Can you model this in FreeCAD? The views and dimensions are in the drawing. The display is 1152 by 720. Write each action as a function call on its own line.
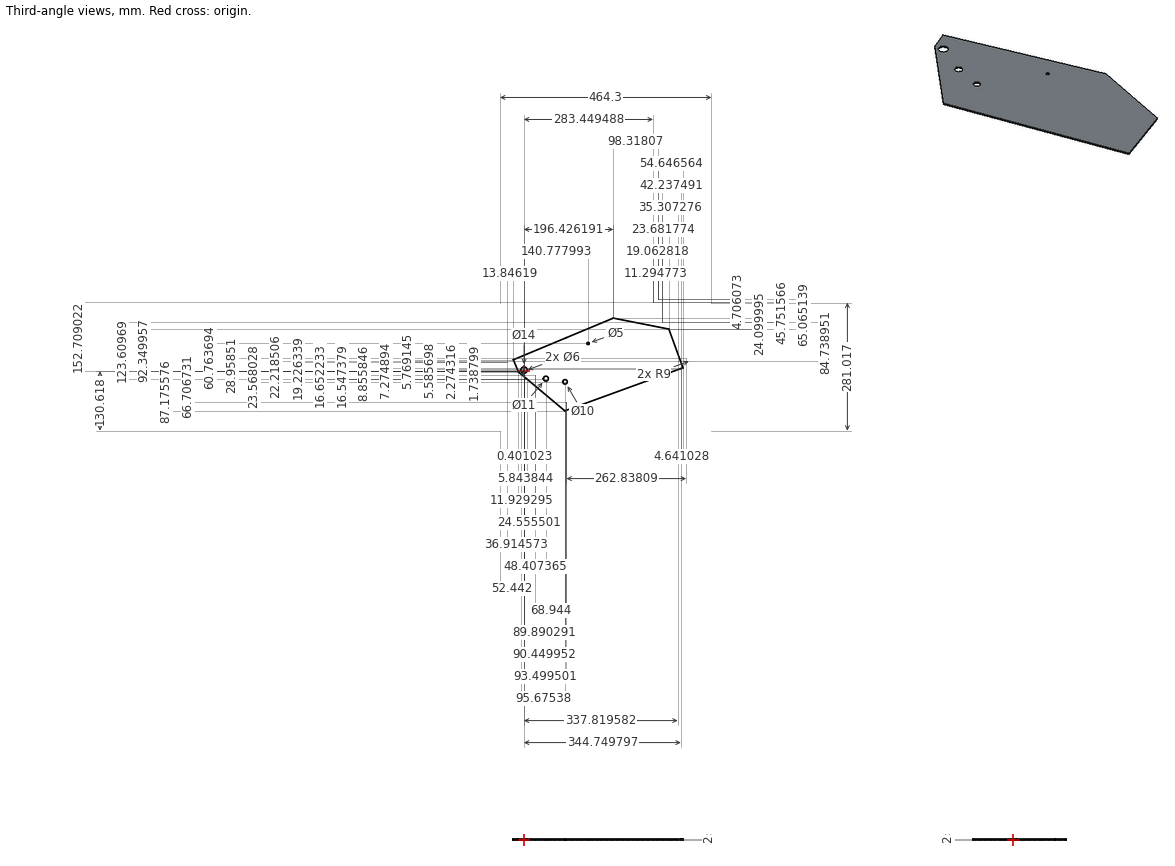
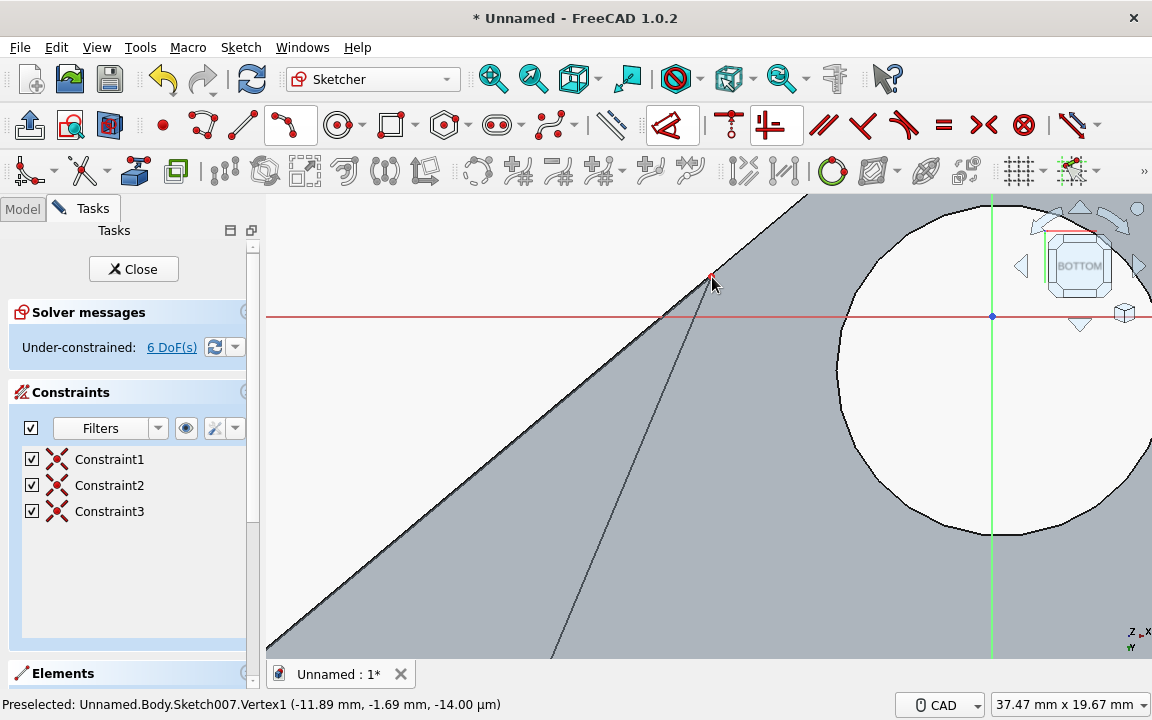
click(711, 277)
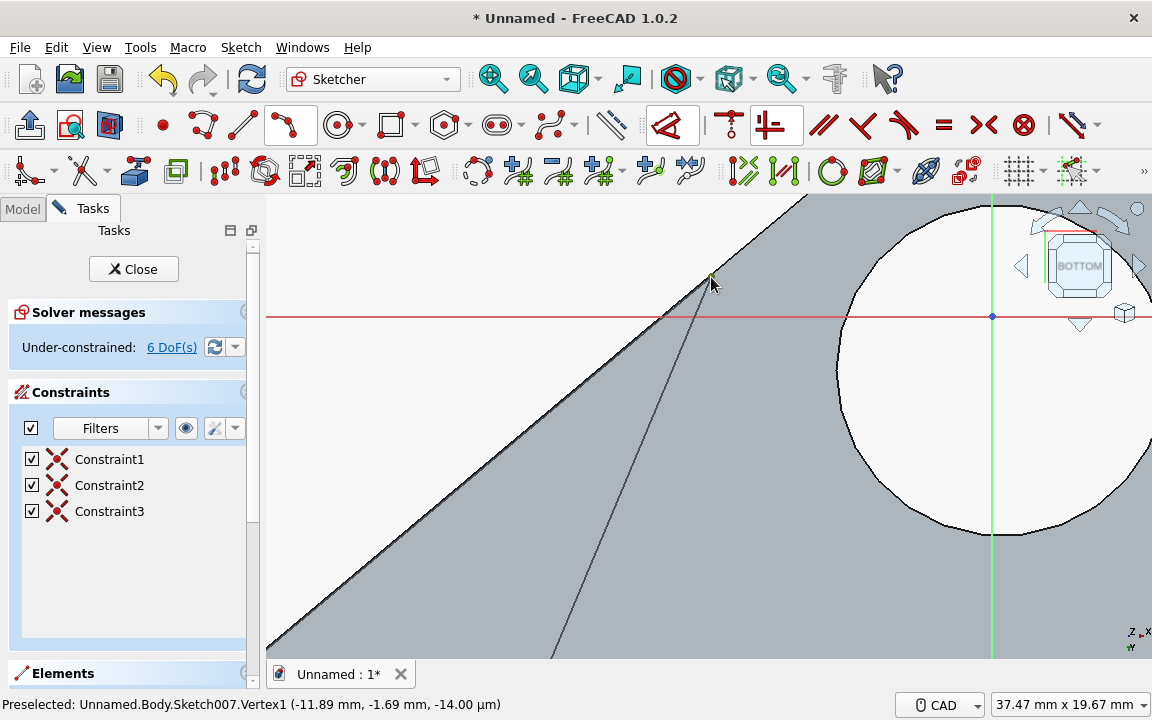
key(i)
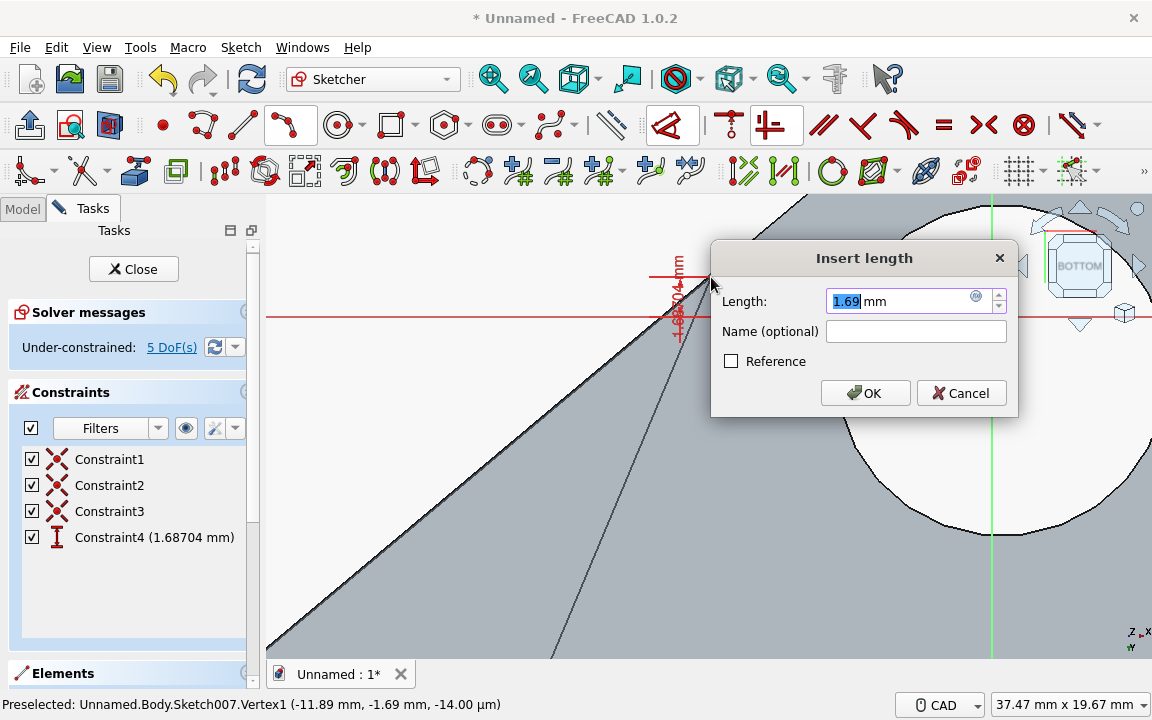
text(1.738799)
key(Return)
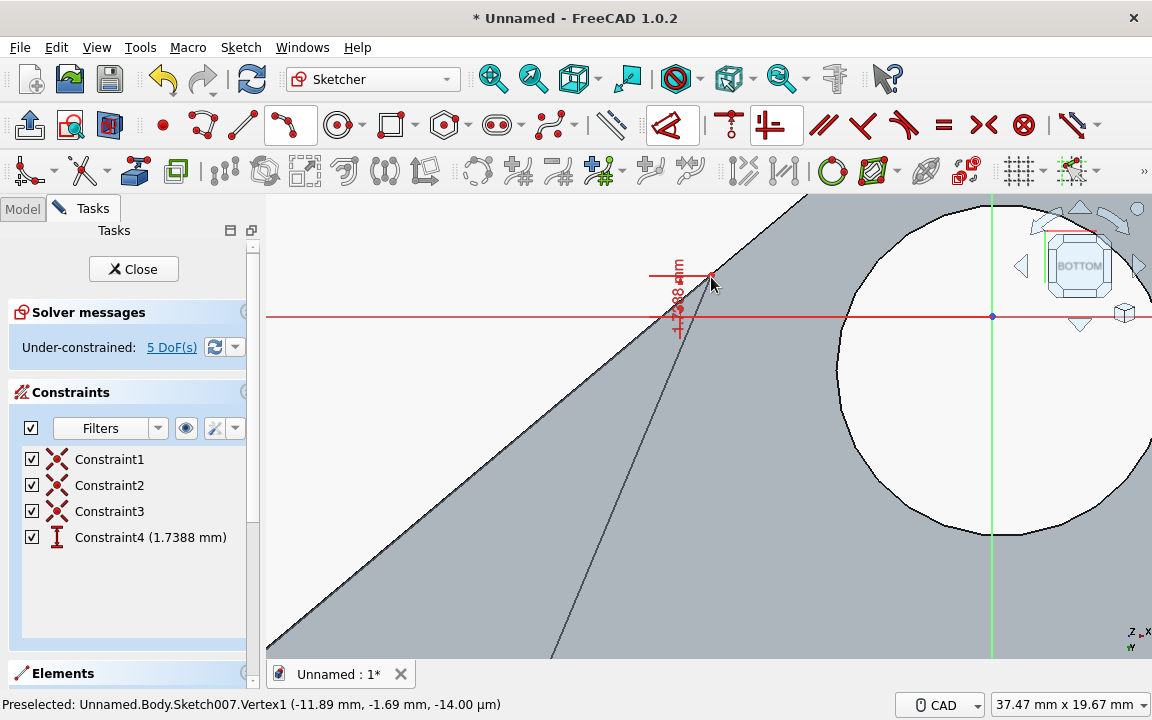
scroll(709, 292, down, 4)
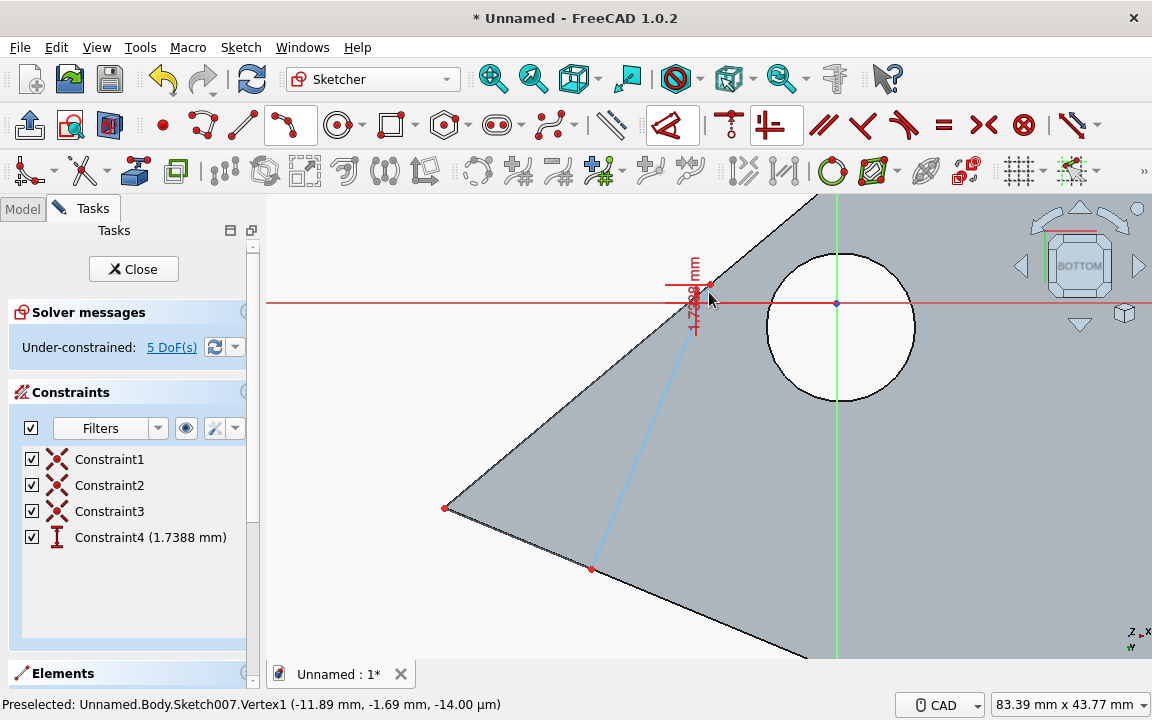
click(488, 527)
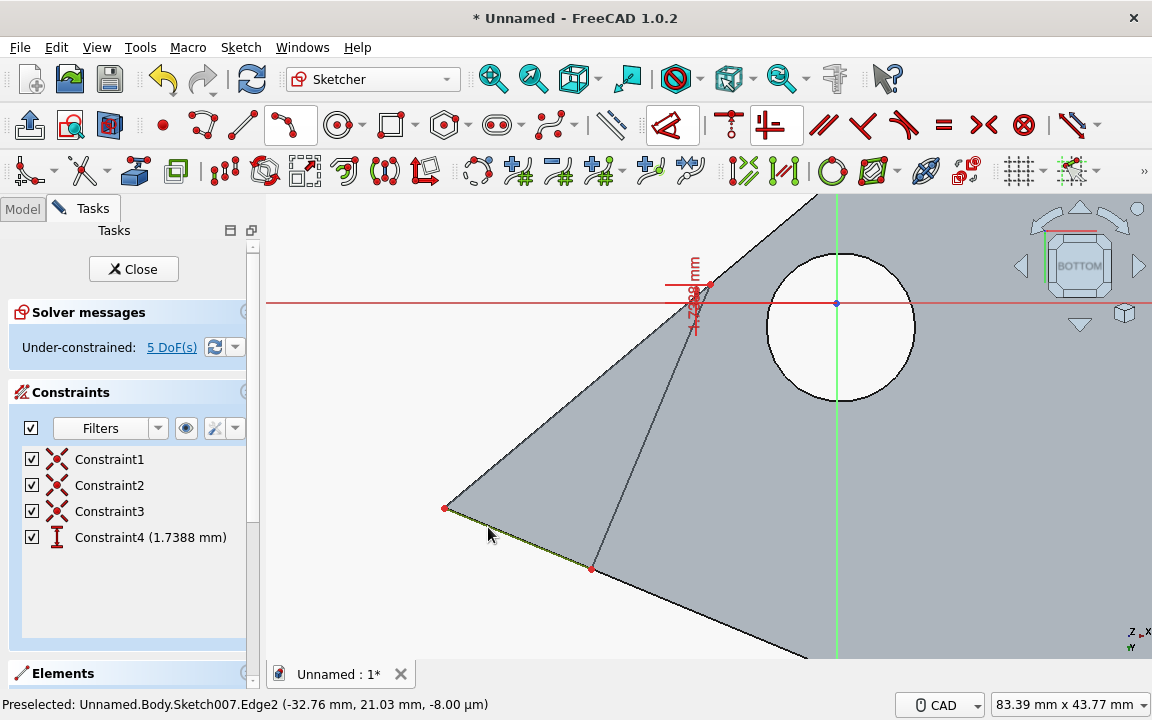
click(694, 126)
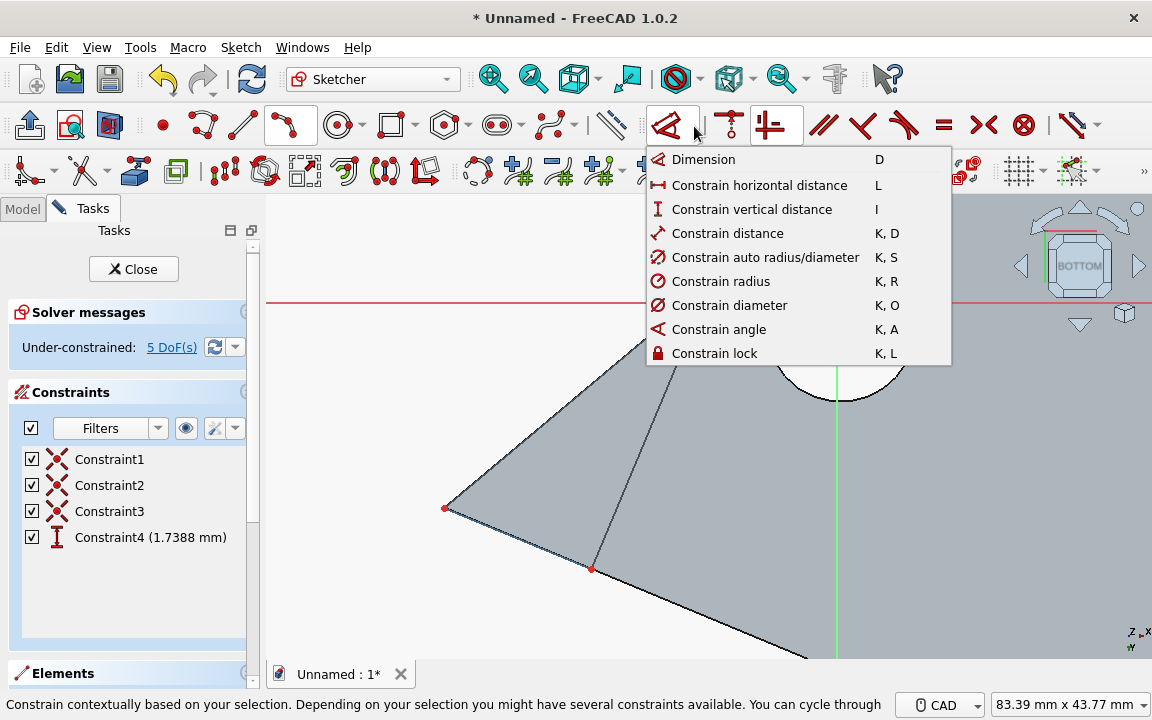
click(799, 185)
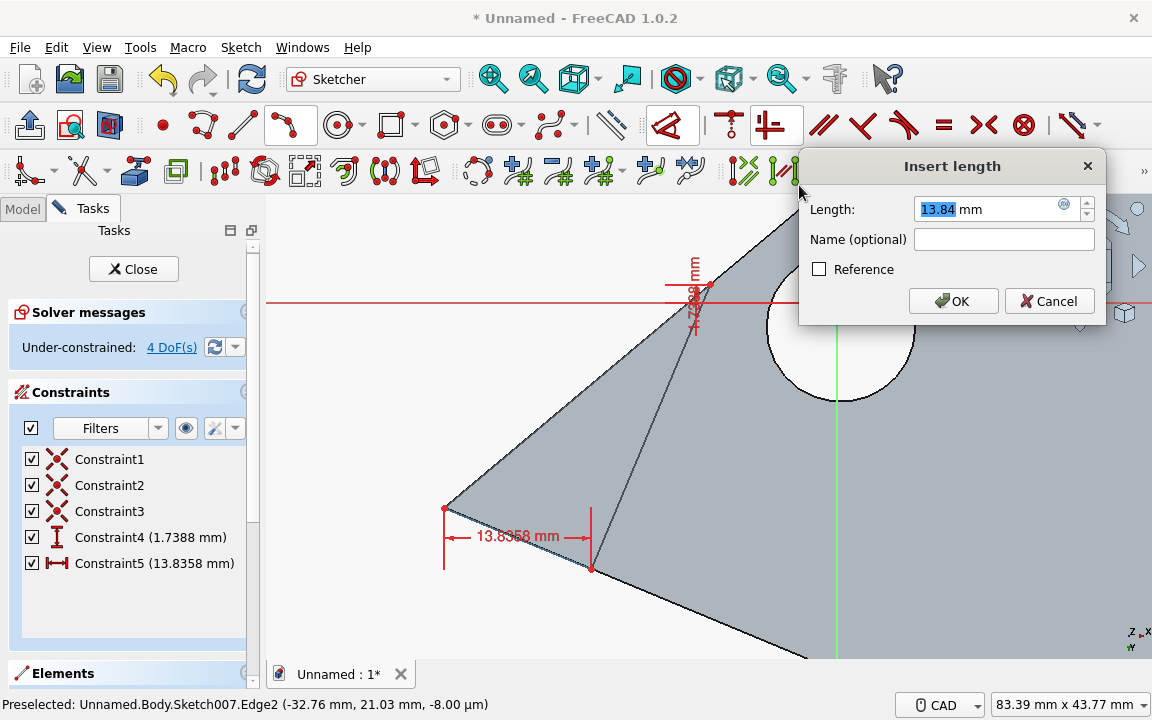
text(13.84619)
key(Return)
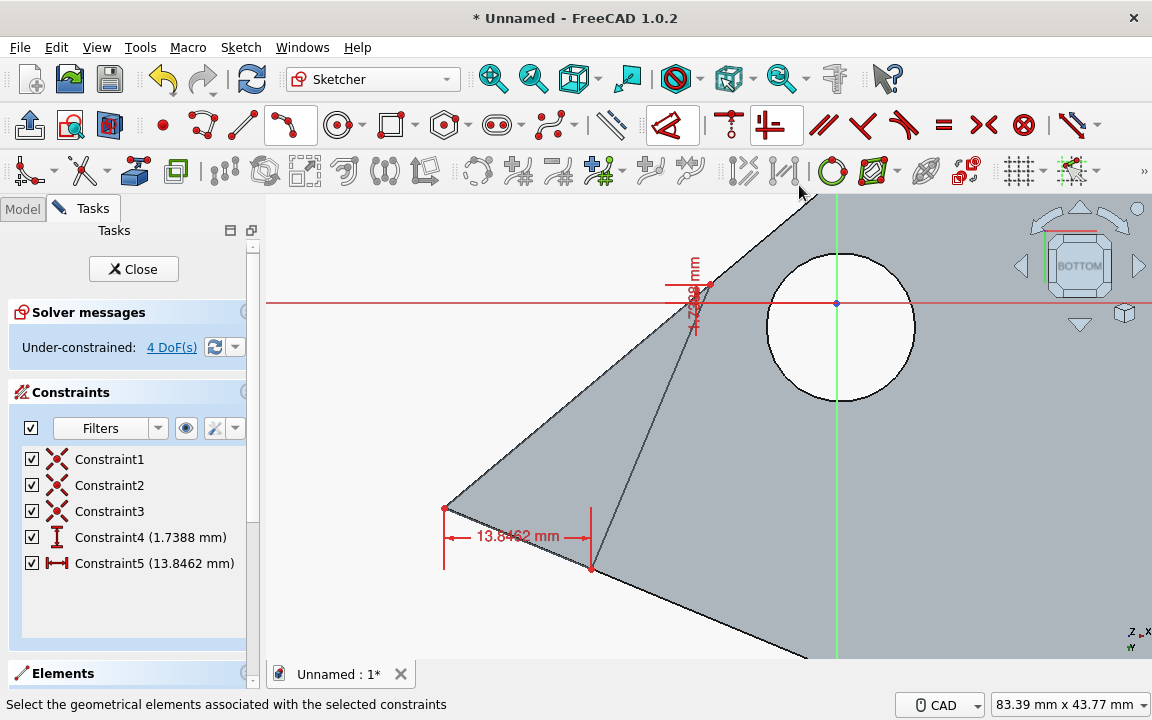
click(488, 527)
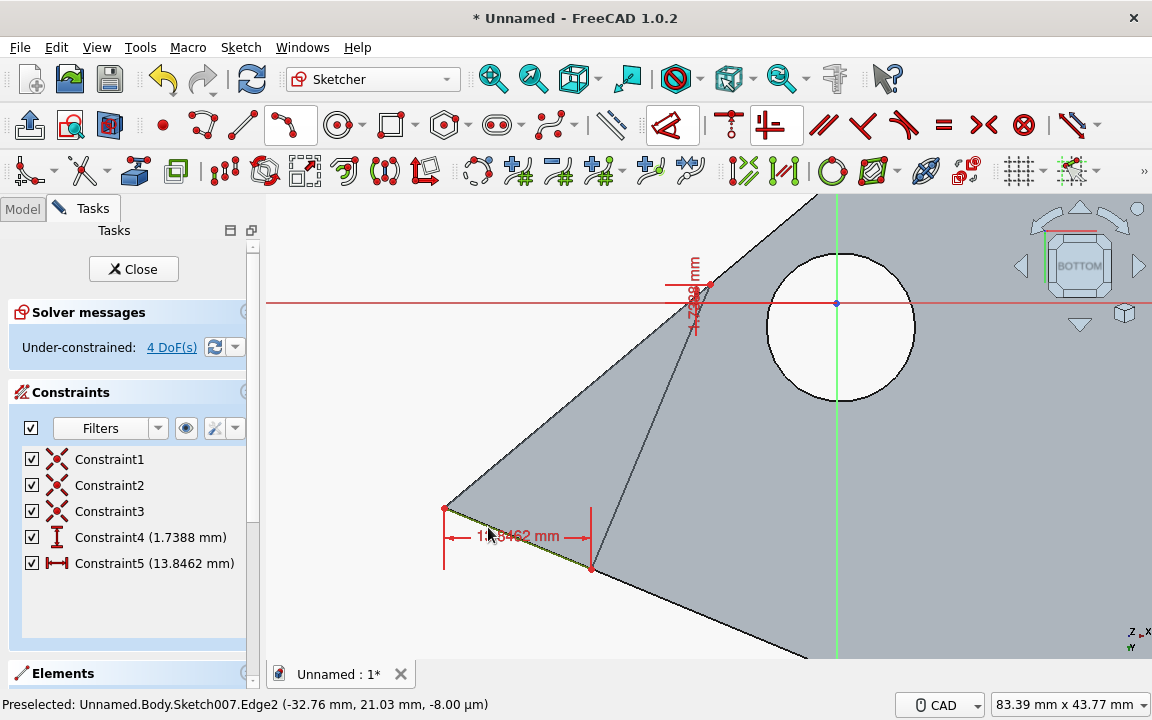
key(i)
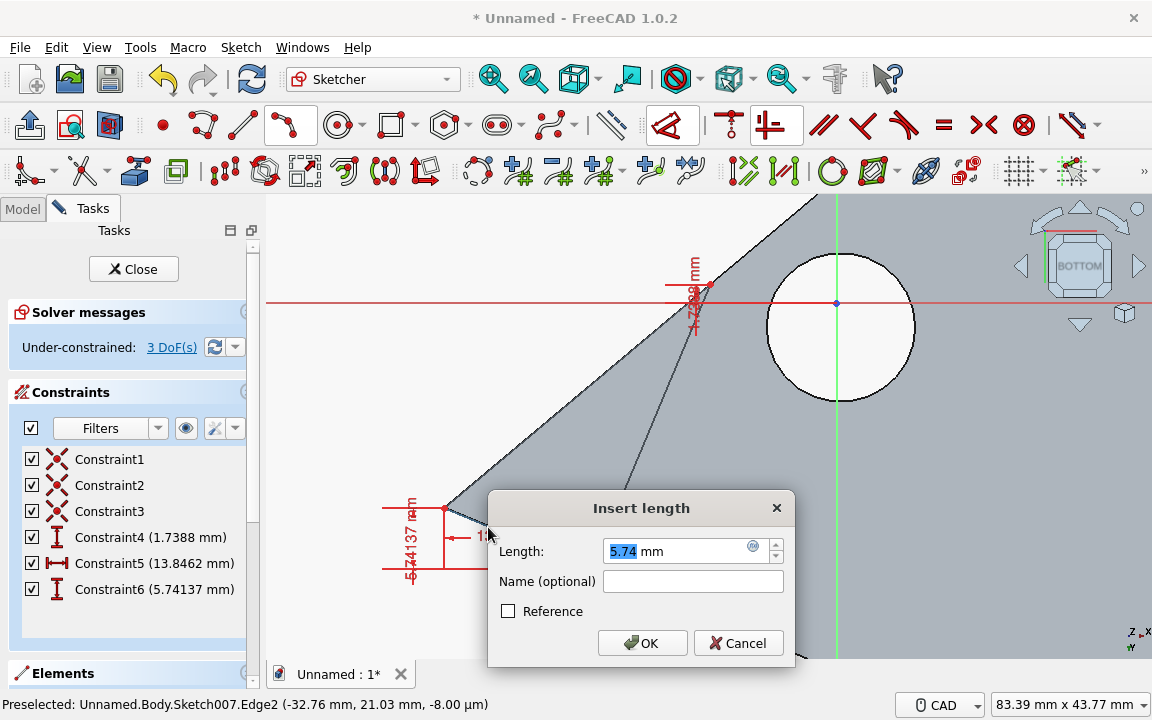
text(5.769145)
key(Return)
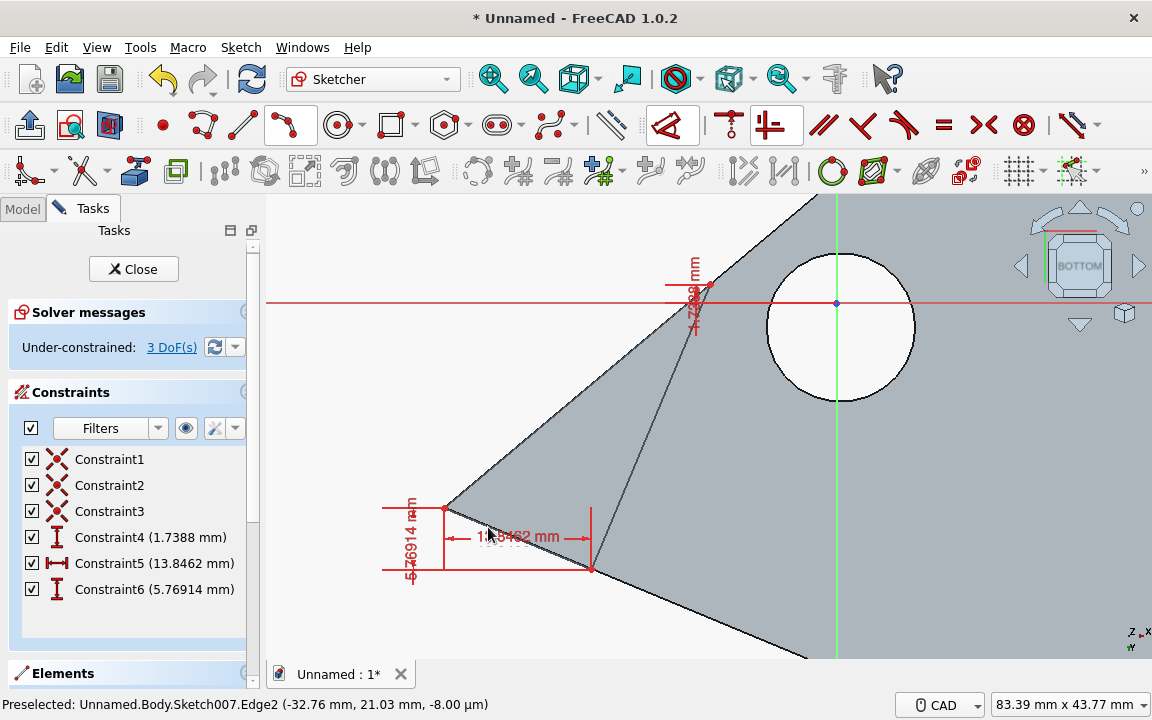
click(710, 285)